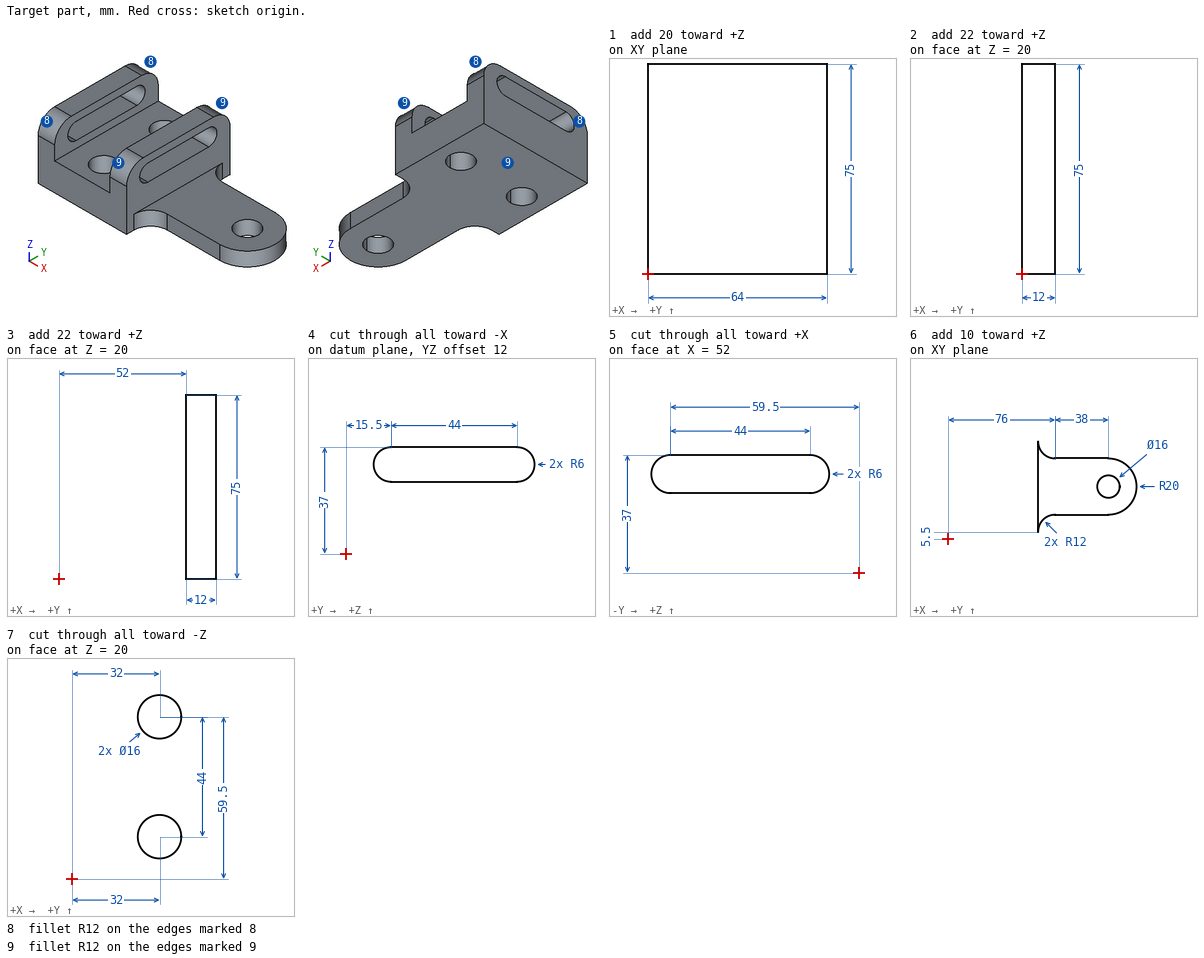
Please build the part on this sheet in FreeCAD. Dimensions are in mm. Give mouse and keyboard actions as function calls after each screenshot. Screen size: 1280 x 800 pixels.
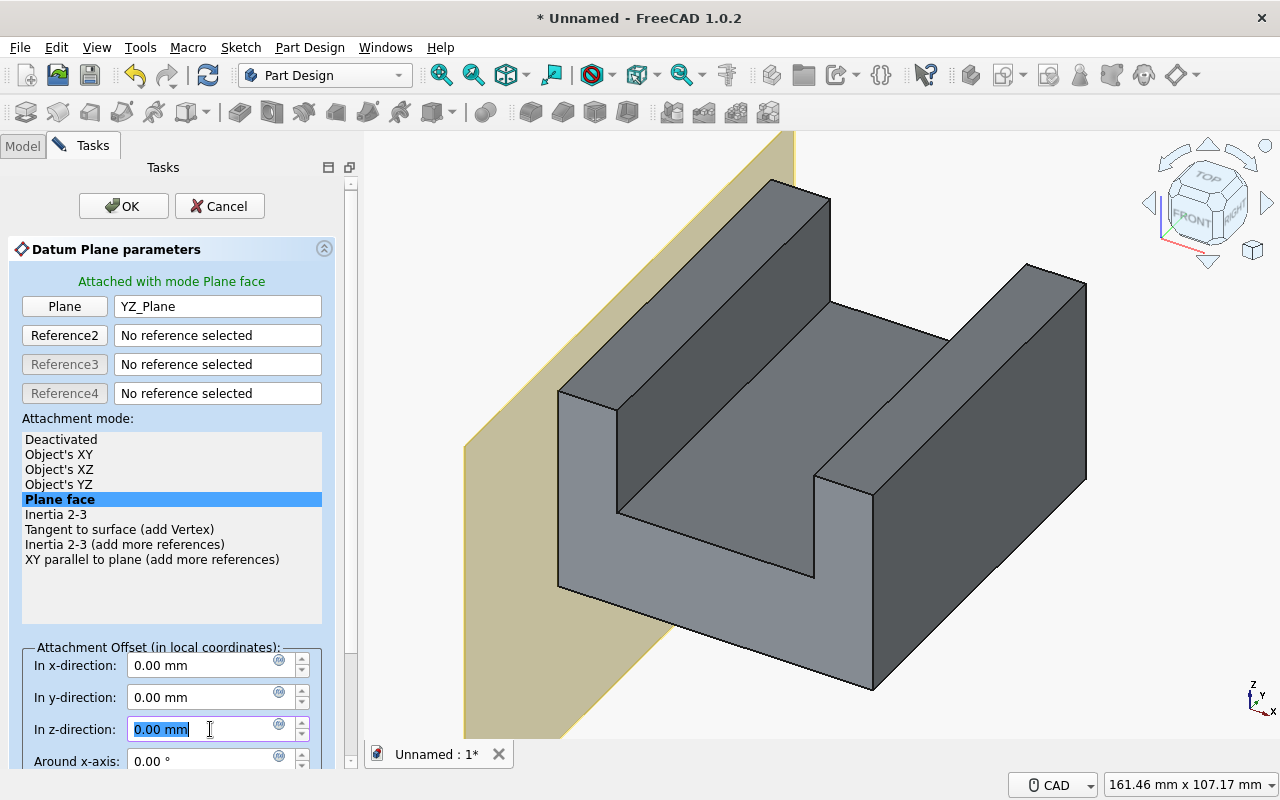
text(12)
key(Tab)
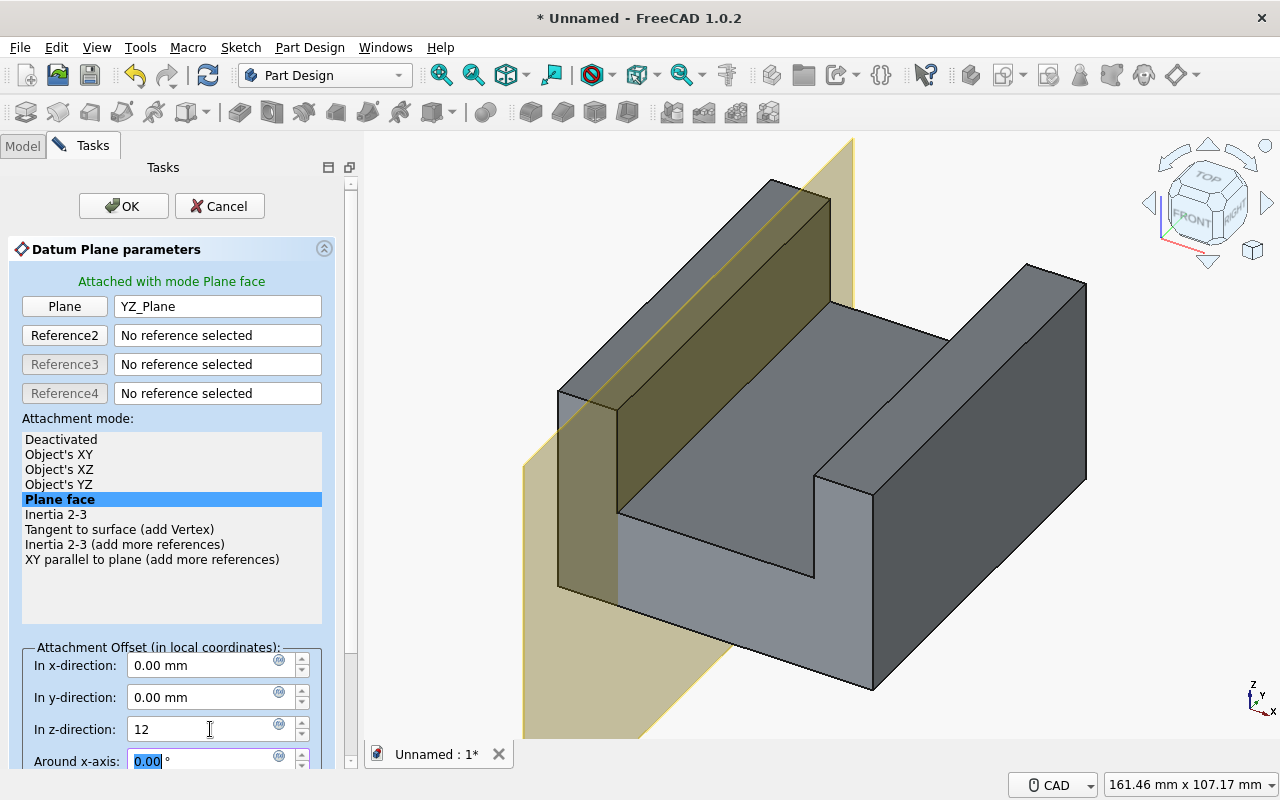
click(124, 206)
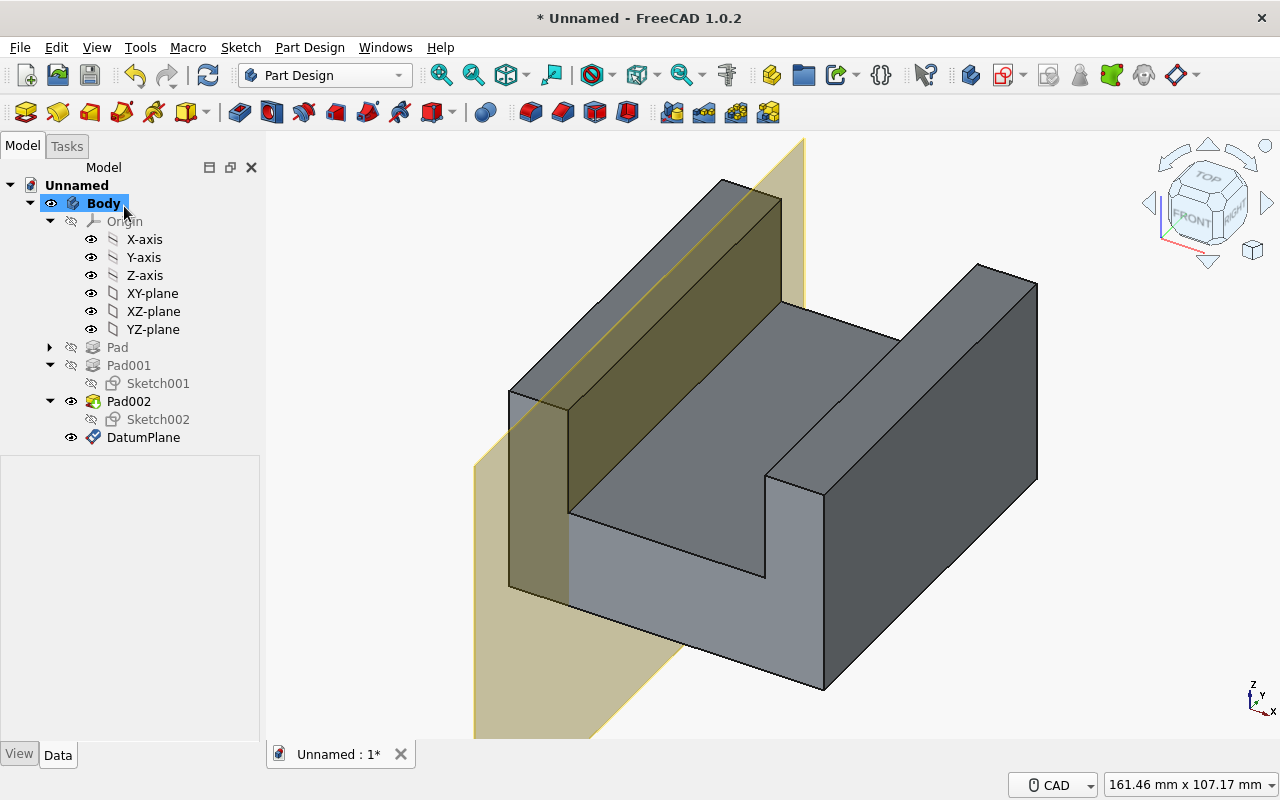
click(116, 437)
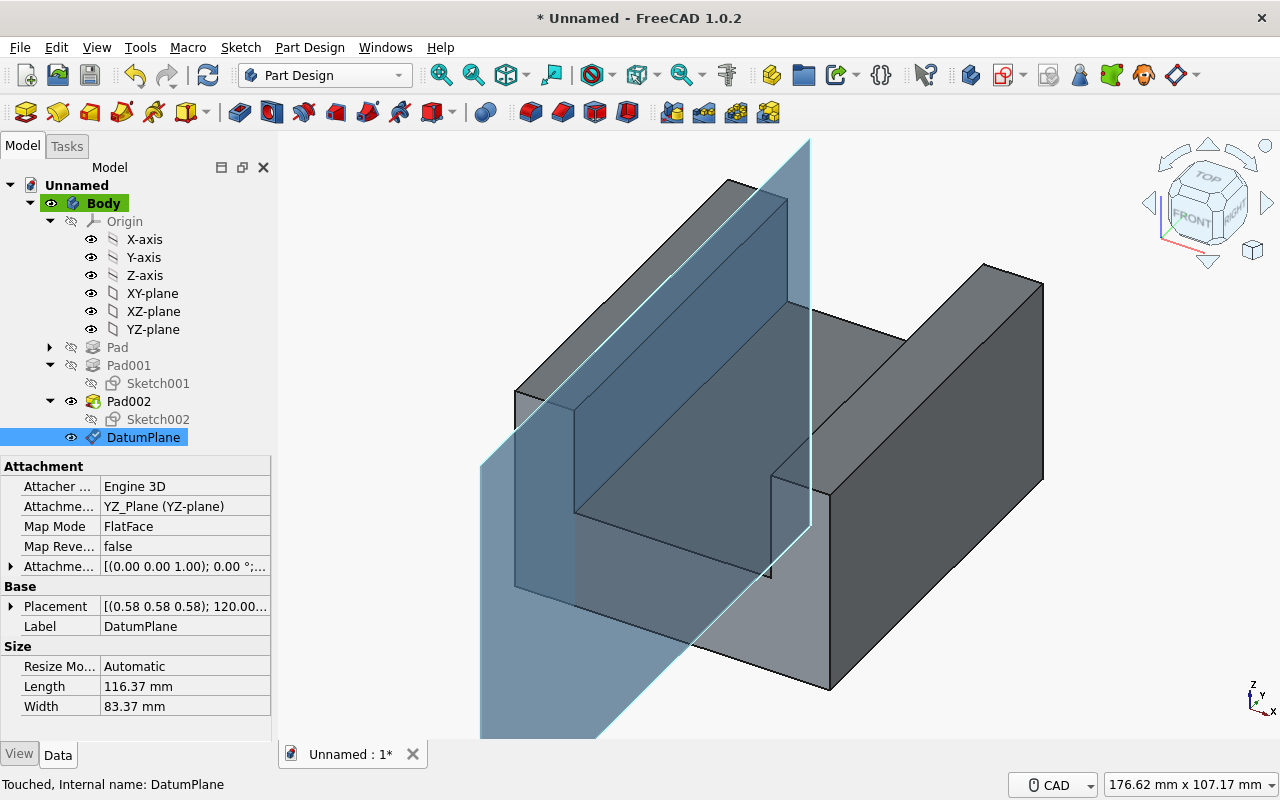
click(1004, 76)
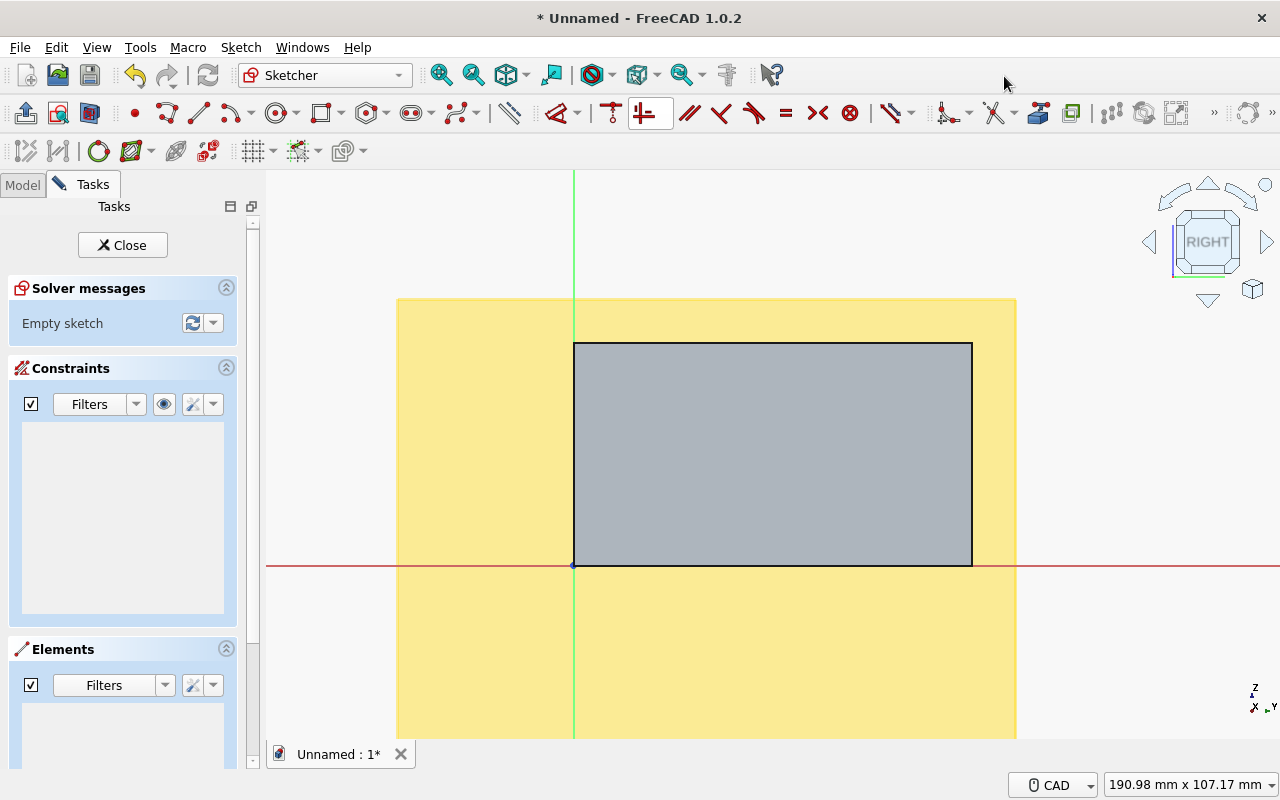
click(90, 114)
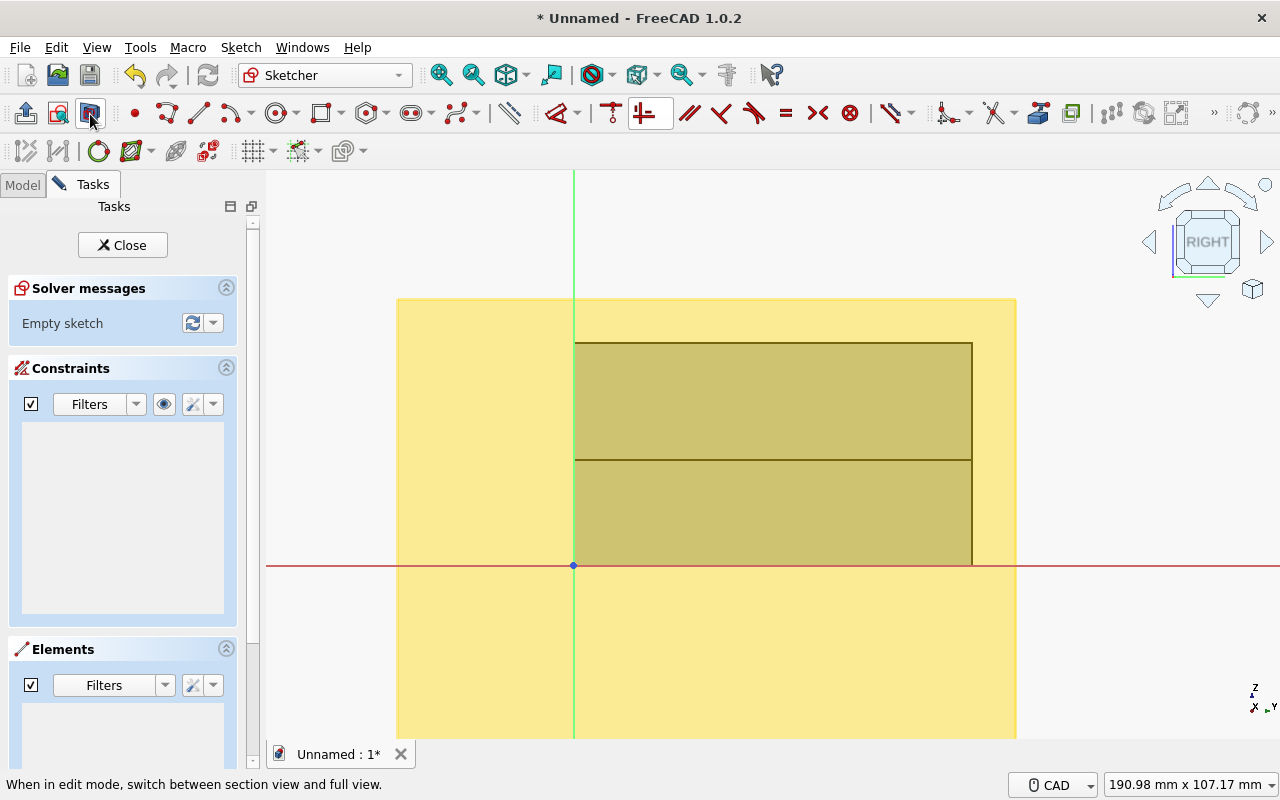
scroll(800, 484, up, 3)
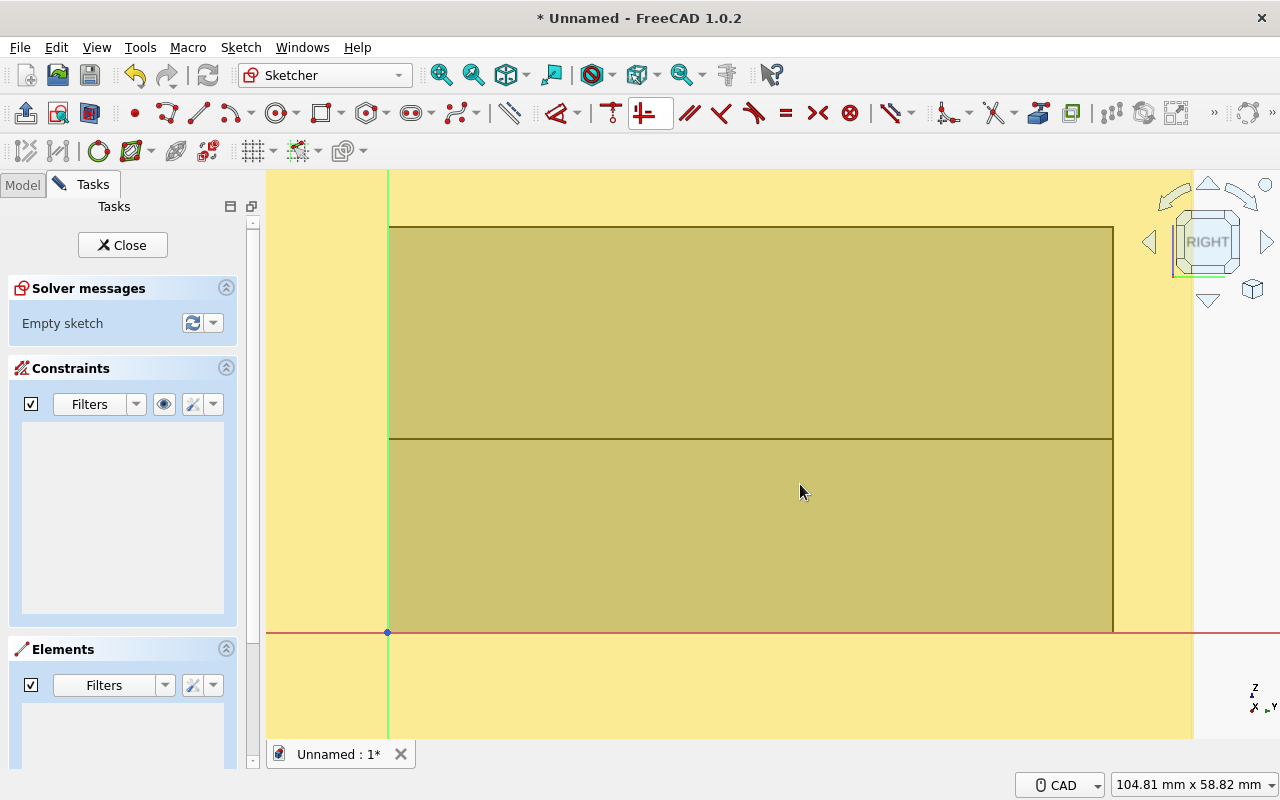
click(412, 114)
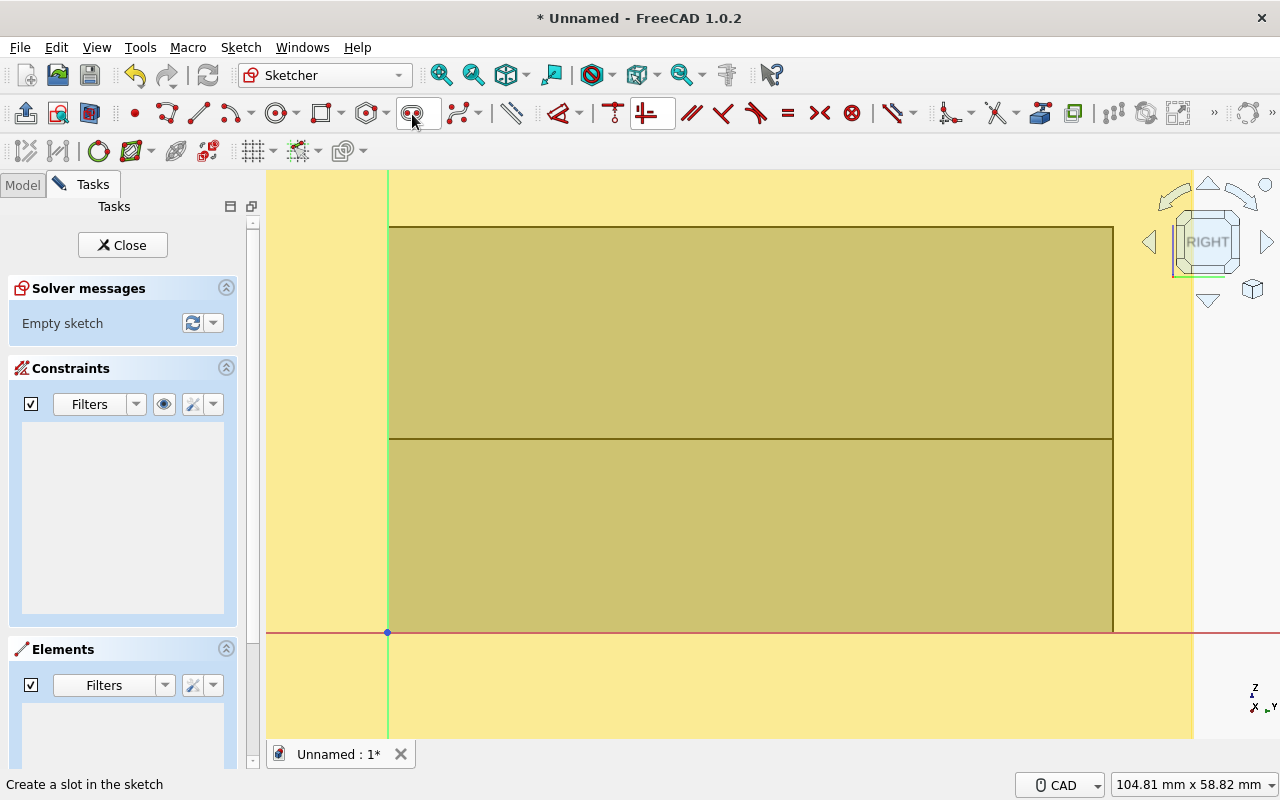
click(538, 333)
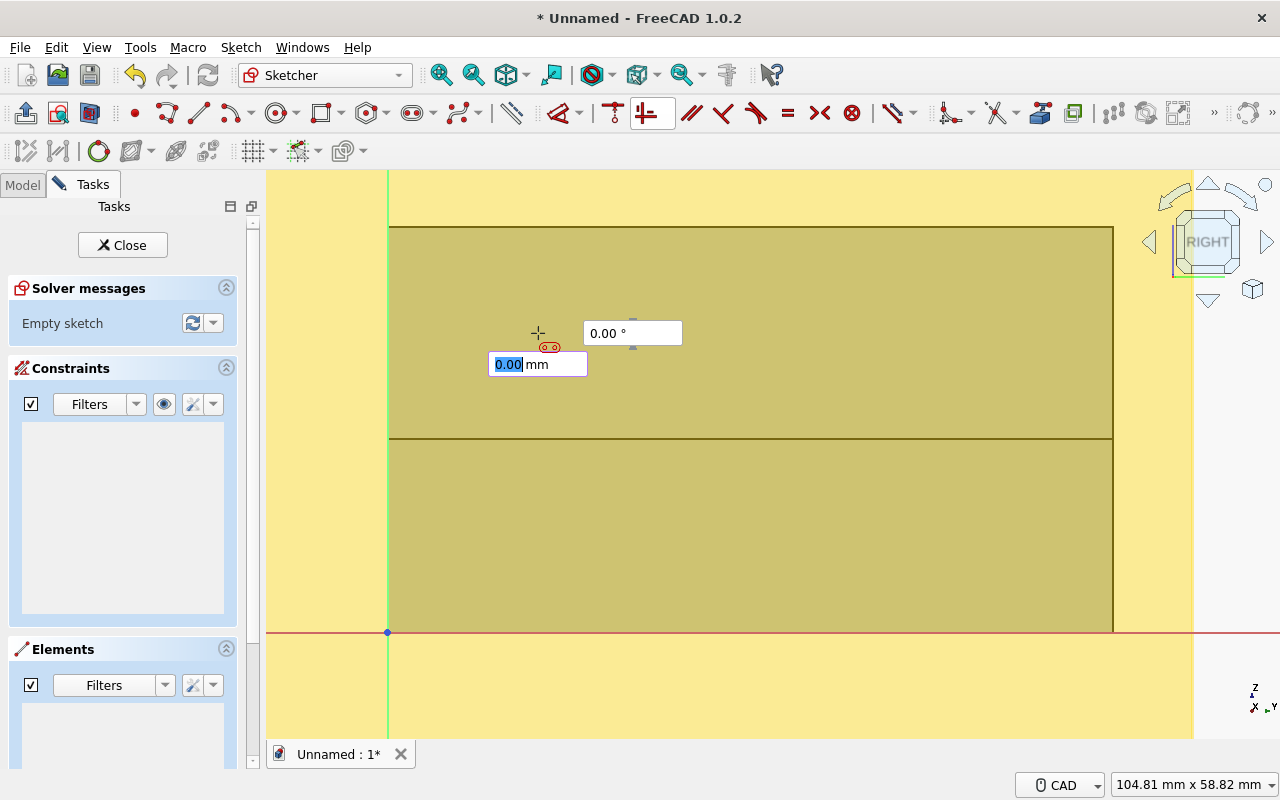
click(963, 333)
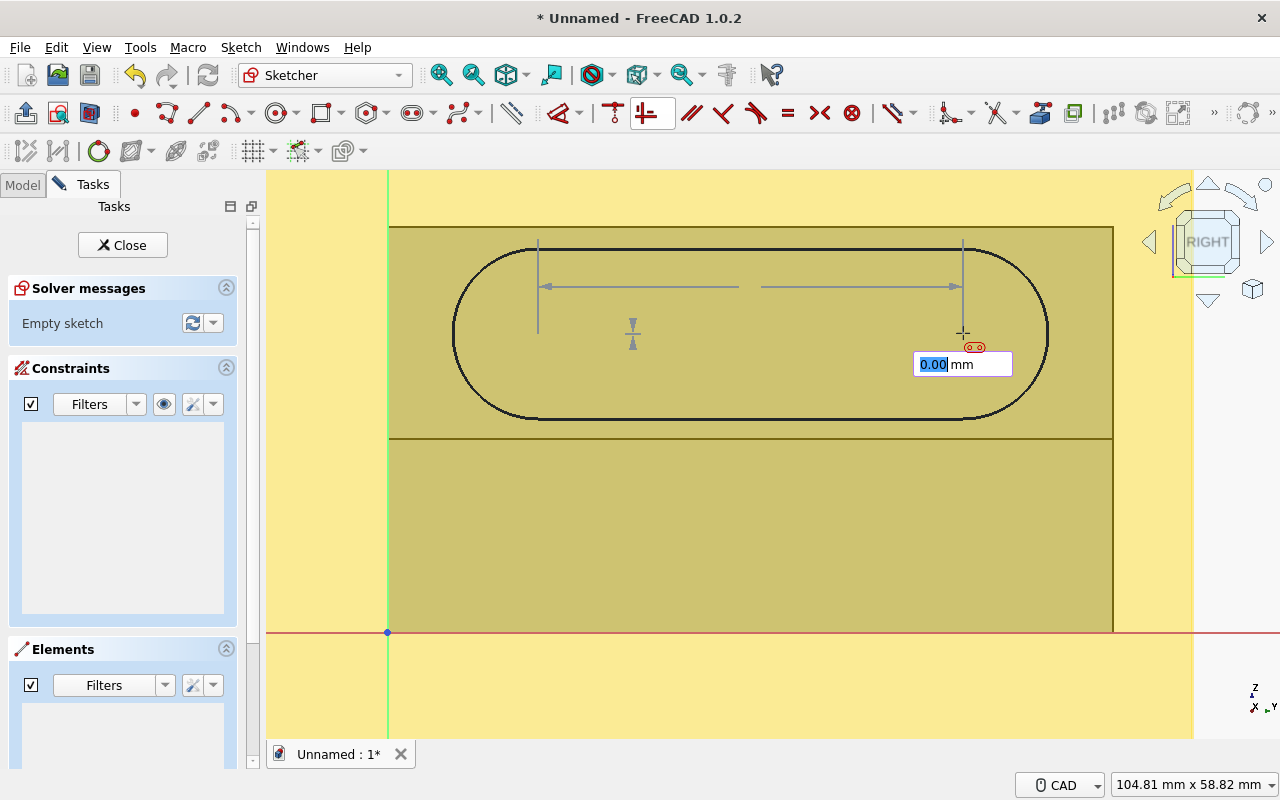
click(750, 275)
key(Escape)